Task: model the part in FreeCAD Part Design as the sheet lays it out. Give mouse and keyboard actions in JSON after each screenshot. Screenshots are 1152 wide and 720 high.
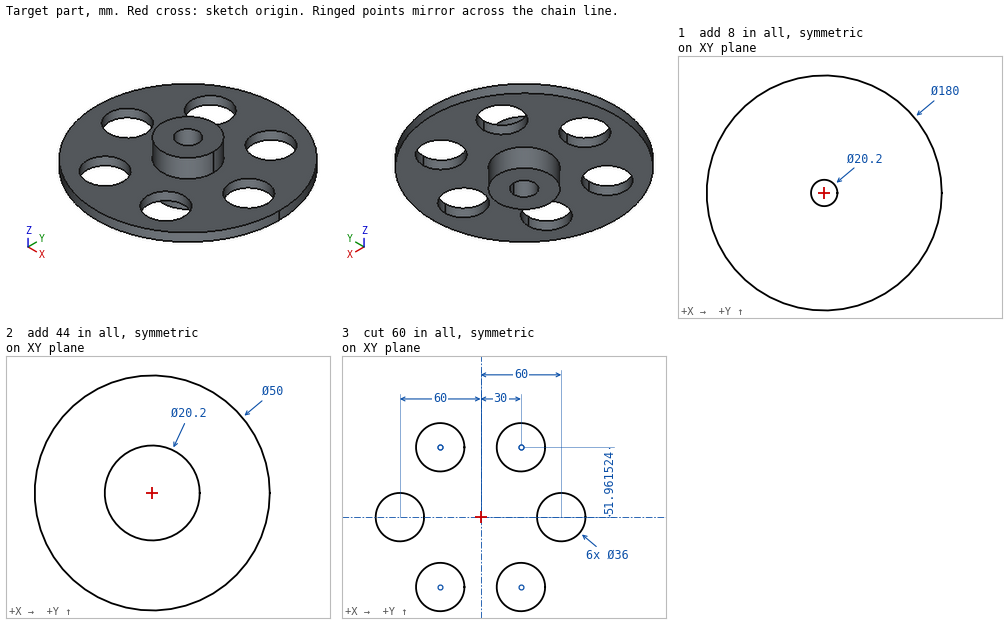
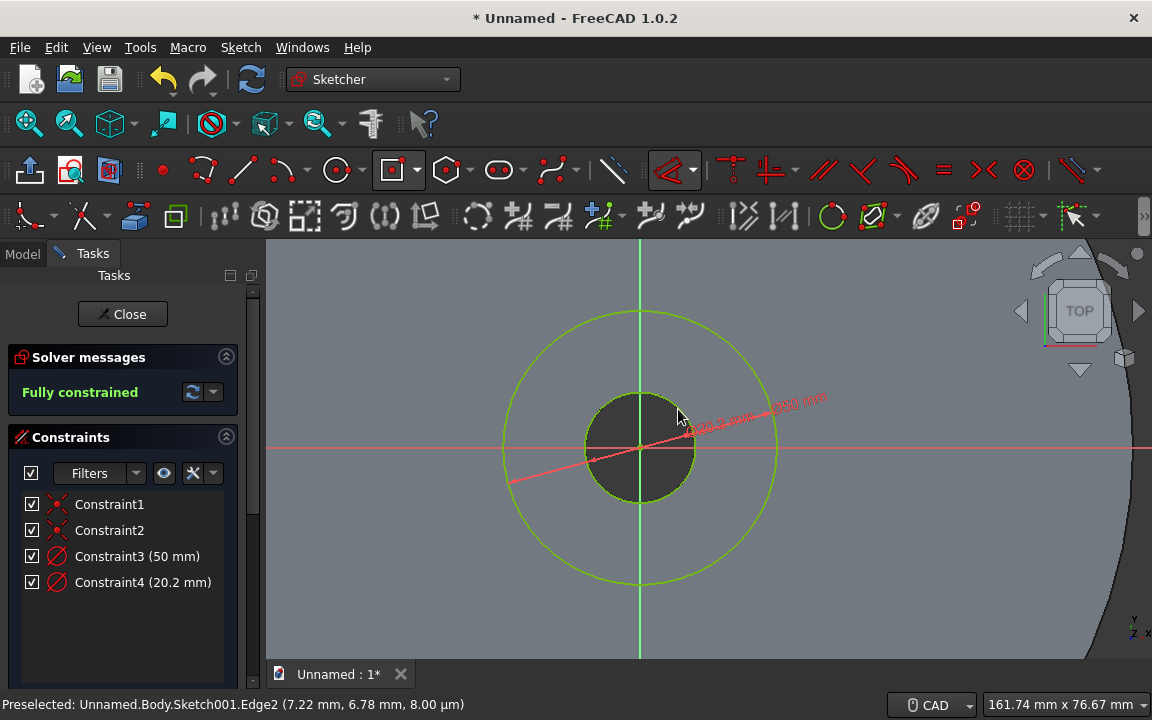
{"action": "left_click", "coordinate": [123, 314]}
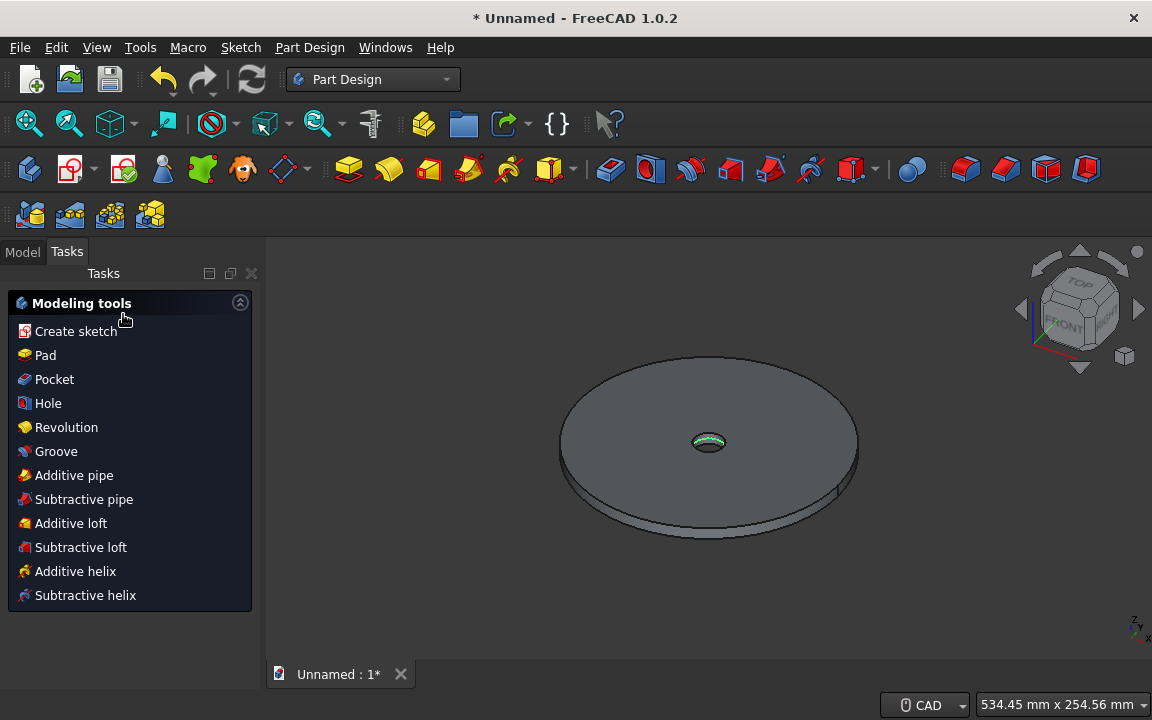
{"action": "left_click", "coordinate": [350, 170]}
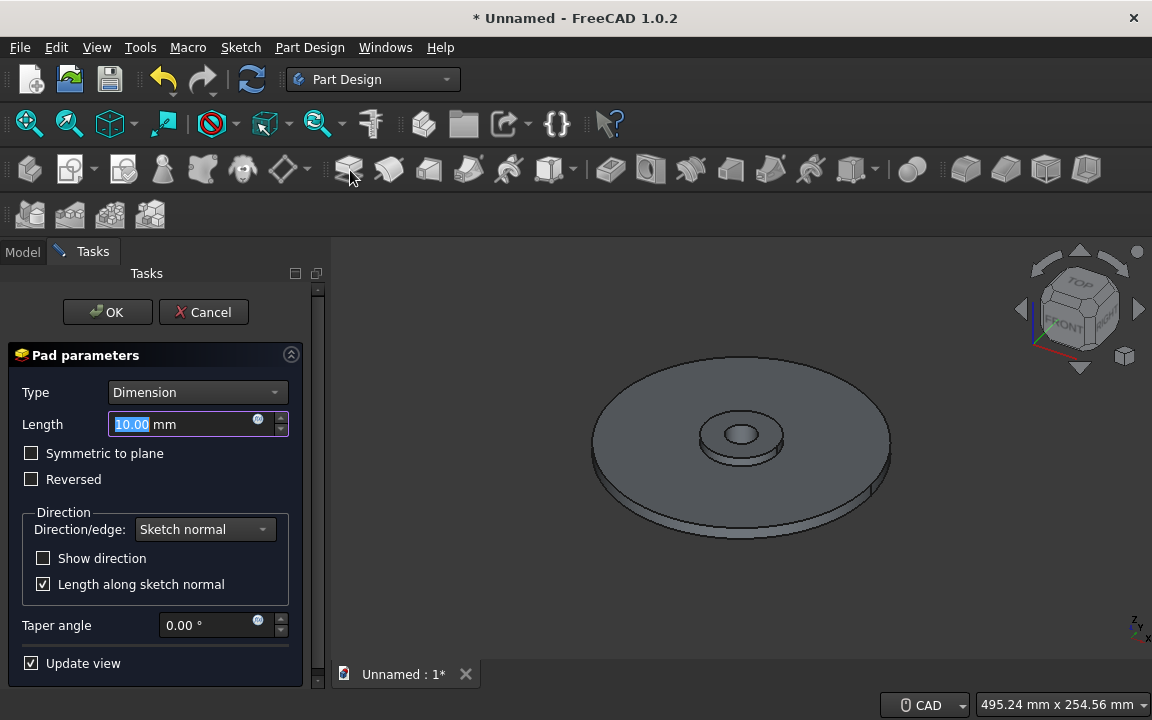
{"action": "type", "text": "44"}
{"action": "key", "text": "Tab"}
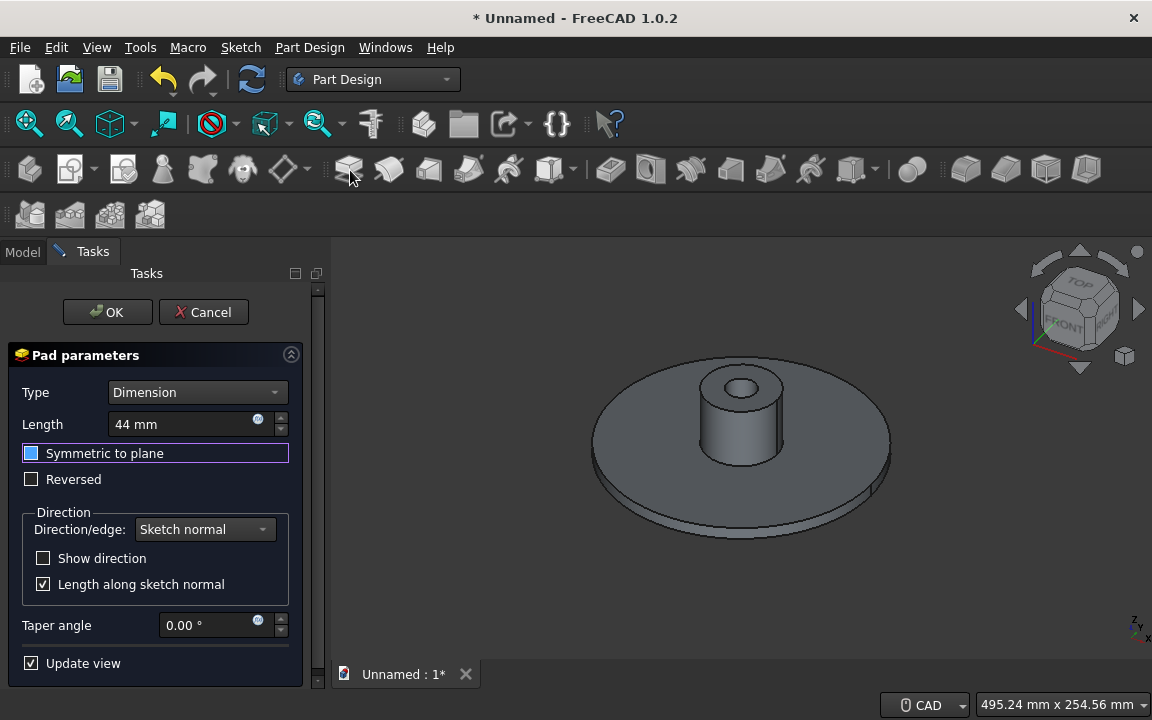
{"action": "left_click", "coordinate": [30, 453]}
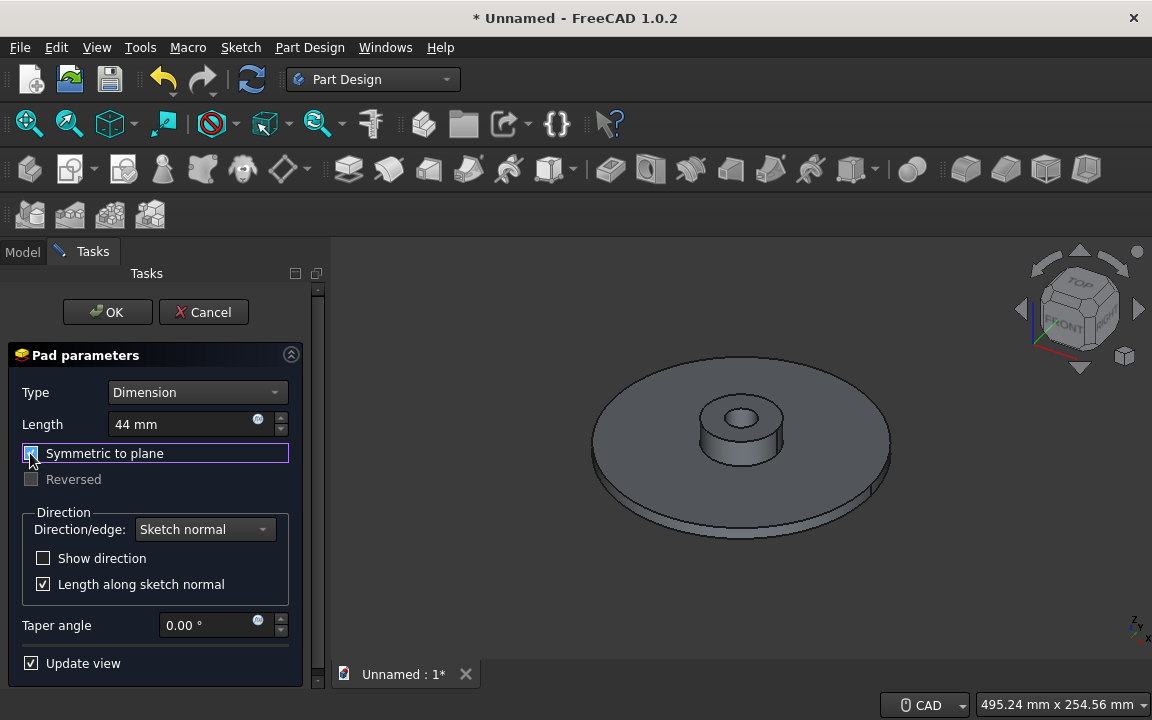
{"action": "left_click", "coordinate": [108, 312]}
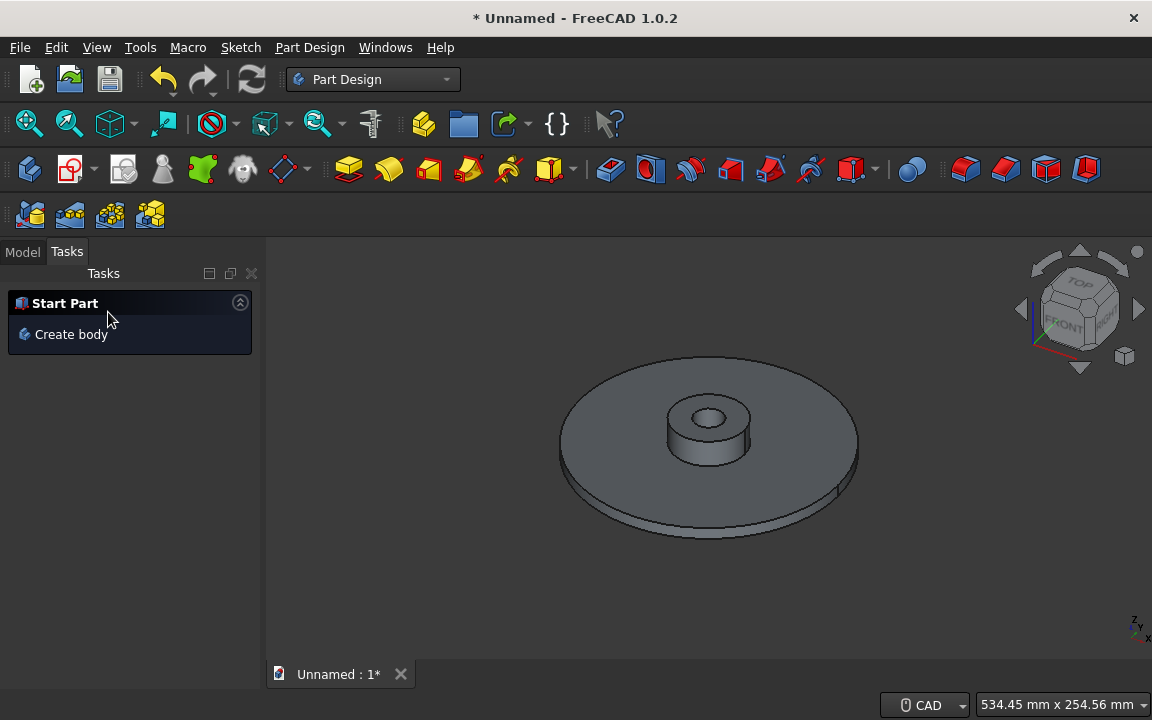
{"action": "left_click", "coordinate": [70, 170]}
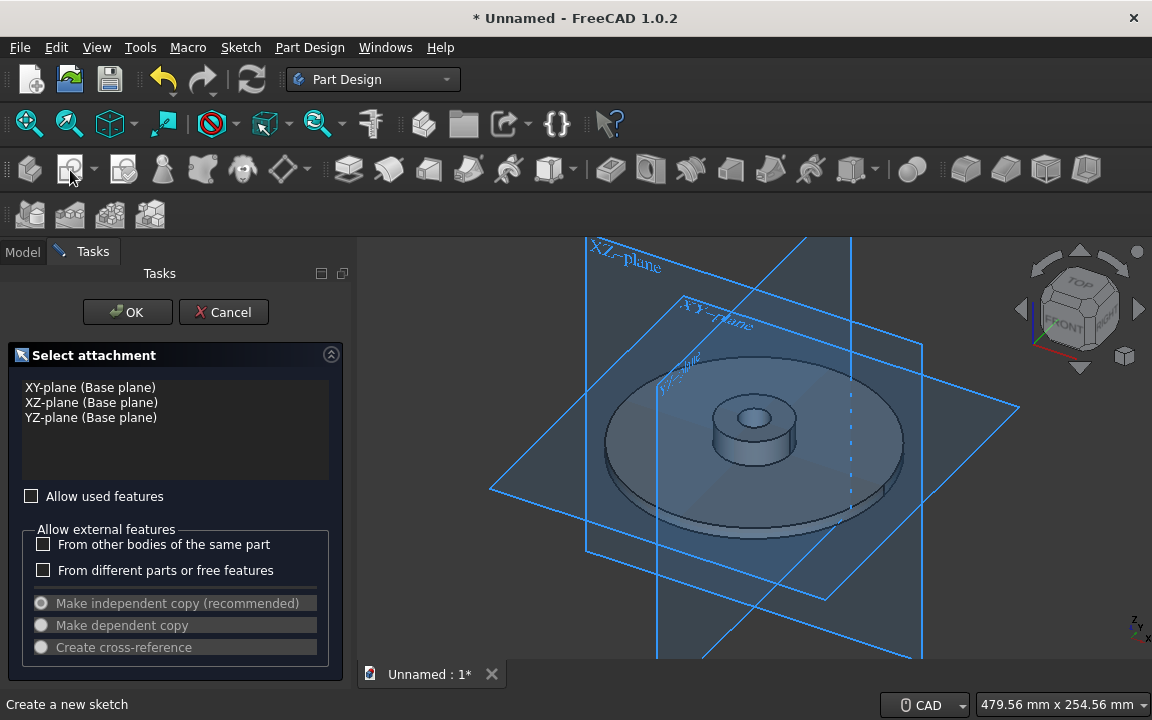
{"action": "left_click", "coordinate": [82, 388]}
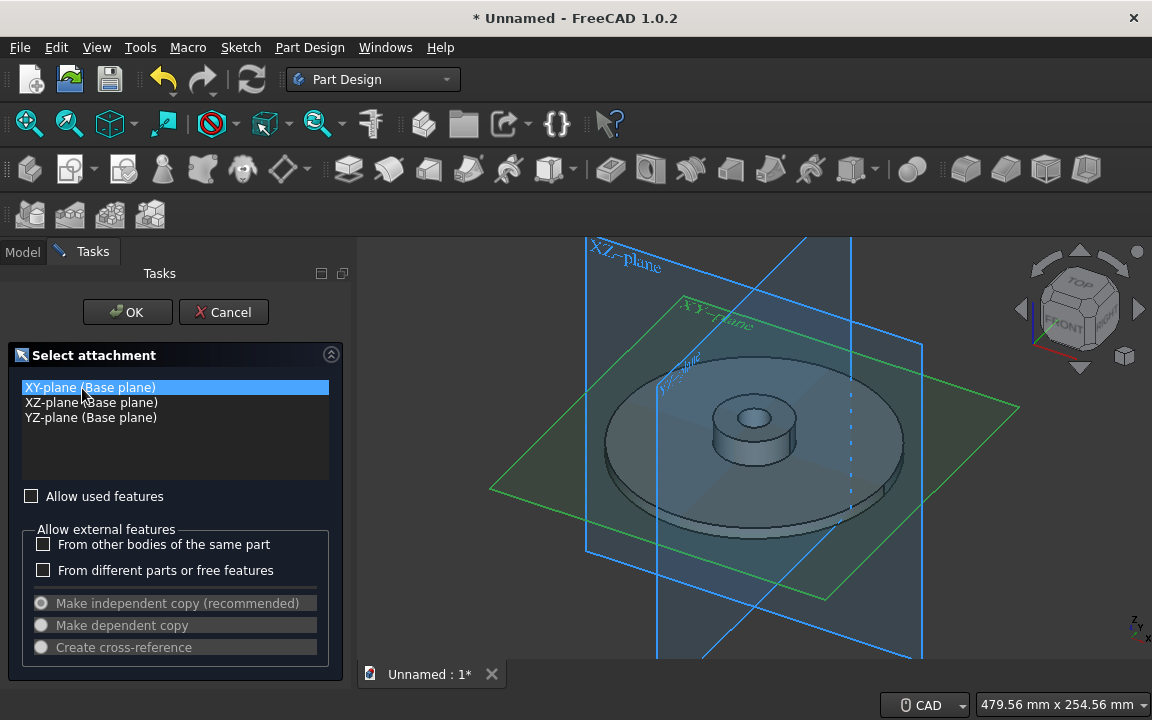
{"action": "left_click", "coordinate": [128, 312]}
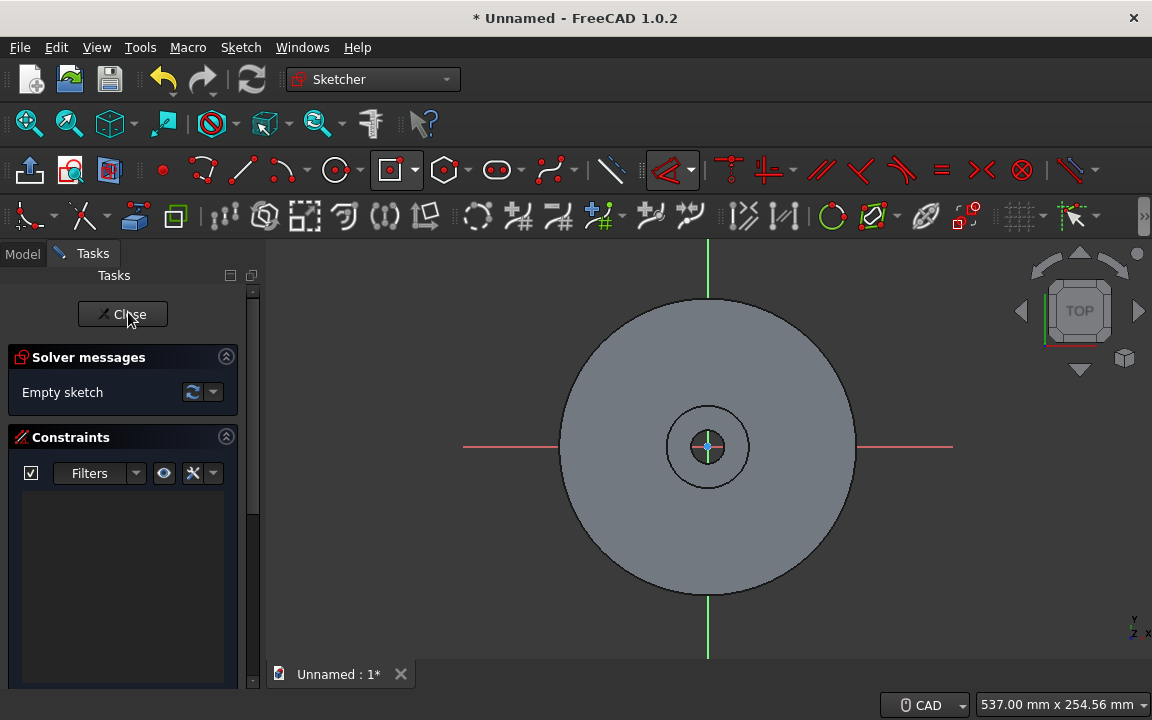
{"action": "key", "text": "q s"}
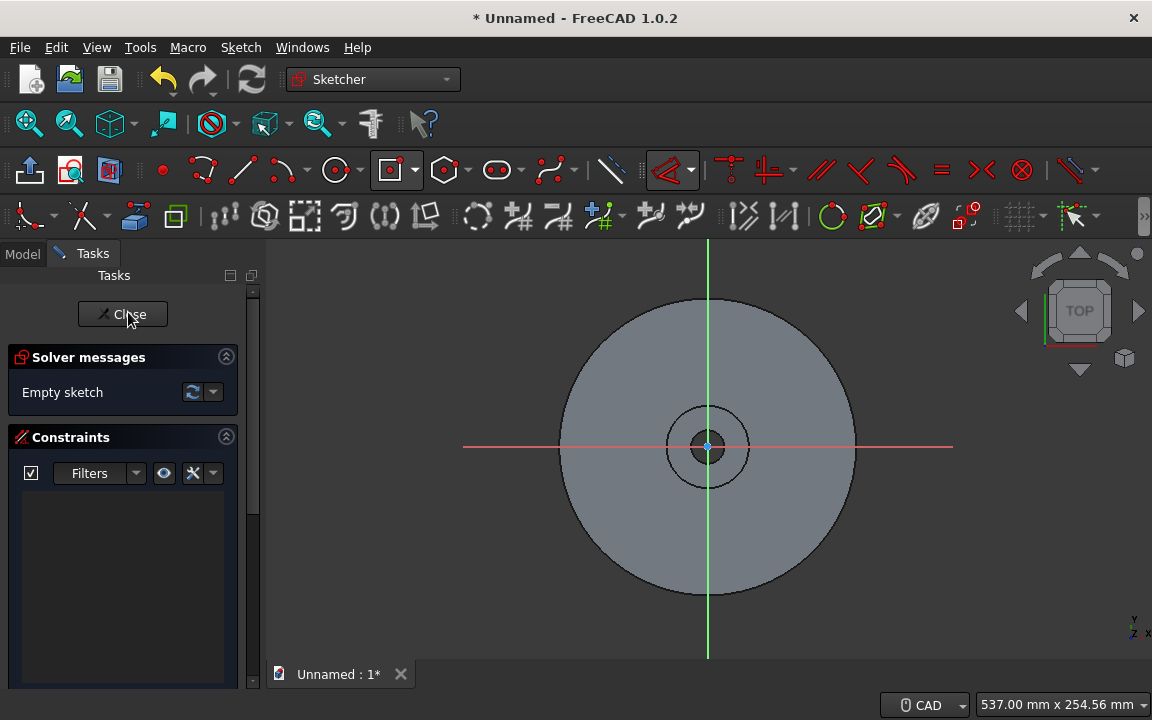
{"action": "left_click", "coordinate": [336, 170]}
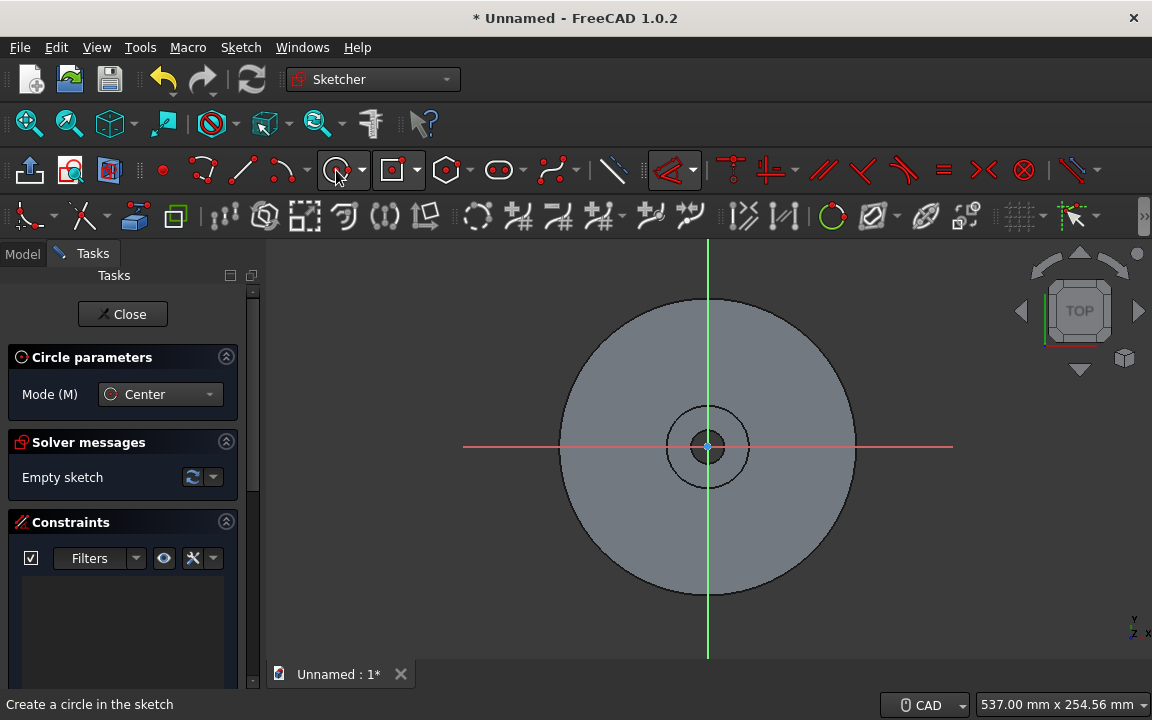
{"action": "left_click", "coordinate": [807, 447]}
{"action": "left_click", "coordinate": [828, 426]}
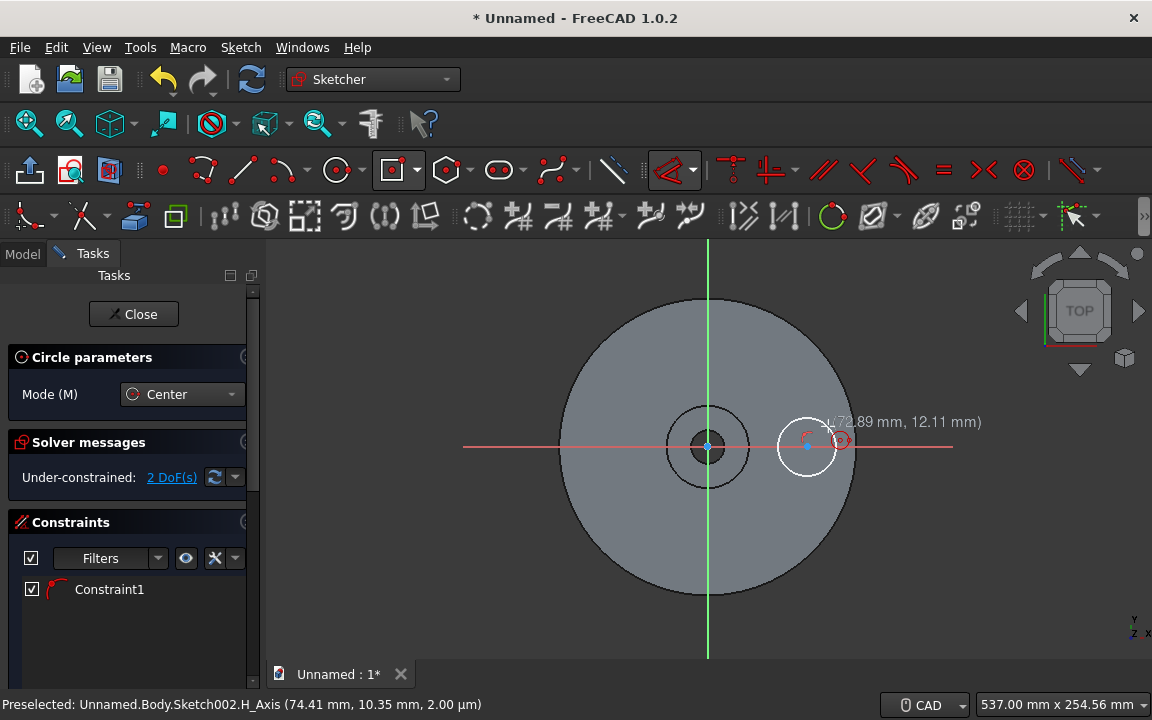
{"action": "left_click", "coordinate": [757, 361]}
{"action": "left_click", "coordinate": [778, 340]}